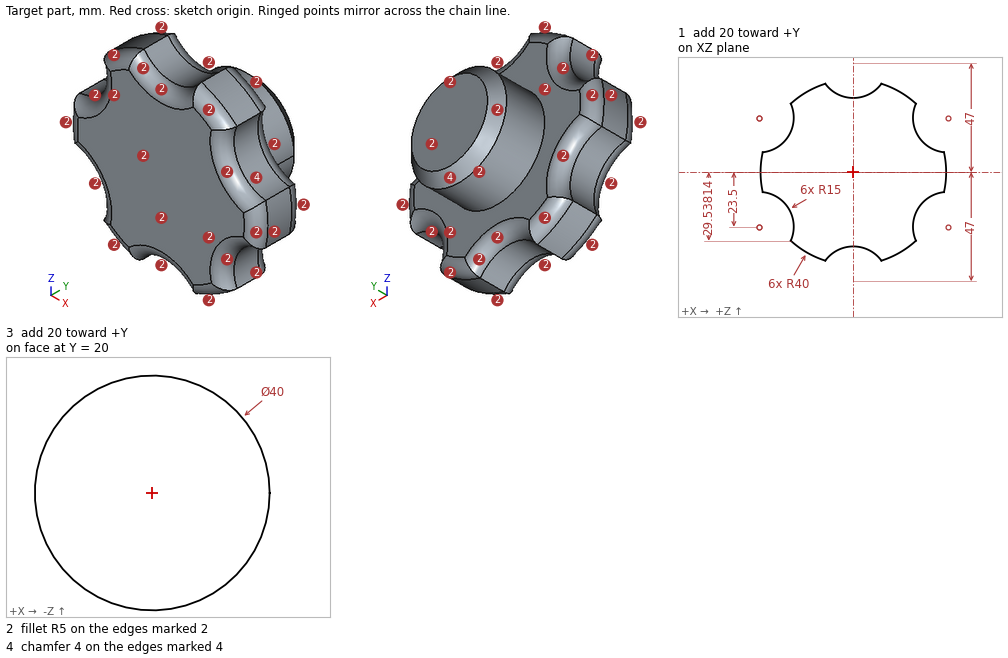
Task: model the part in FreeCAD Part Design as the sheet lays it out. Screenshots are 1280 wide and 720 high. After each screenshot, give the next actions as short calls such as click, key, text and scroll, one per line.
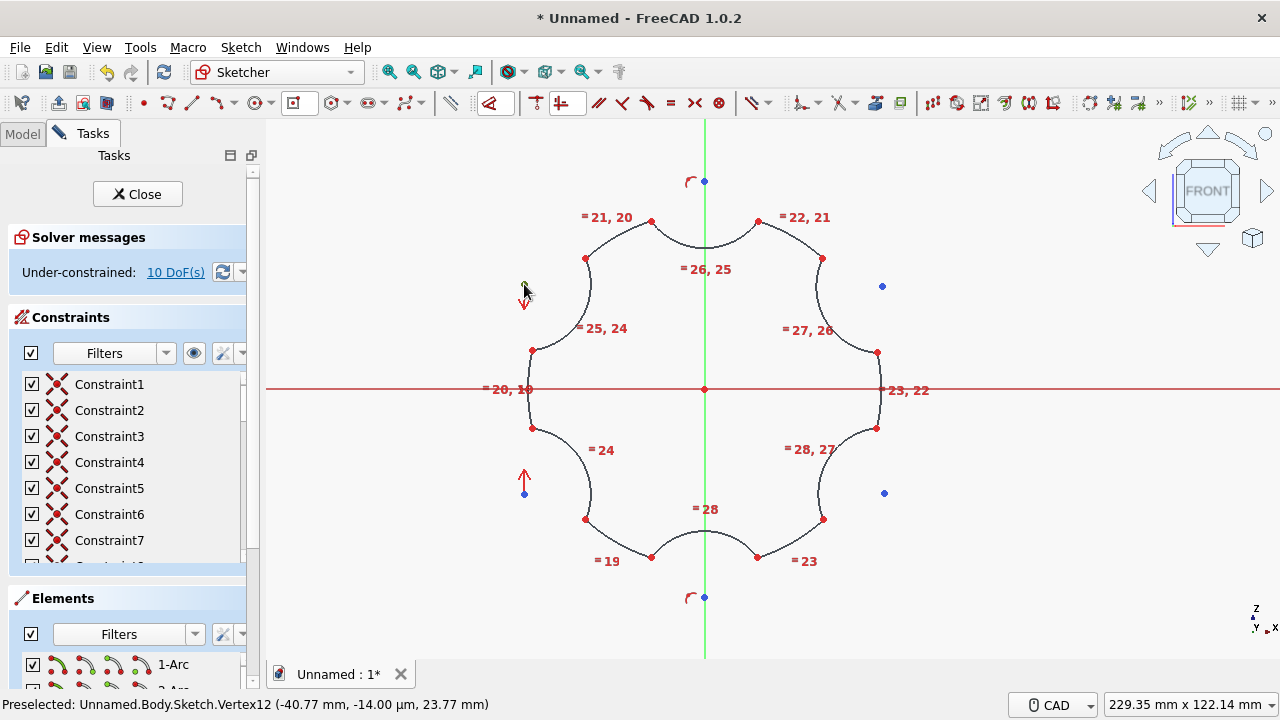
click(883, 287)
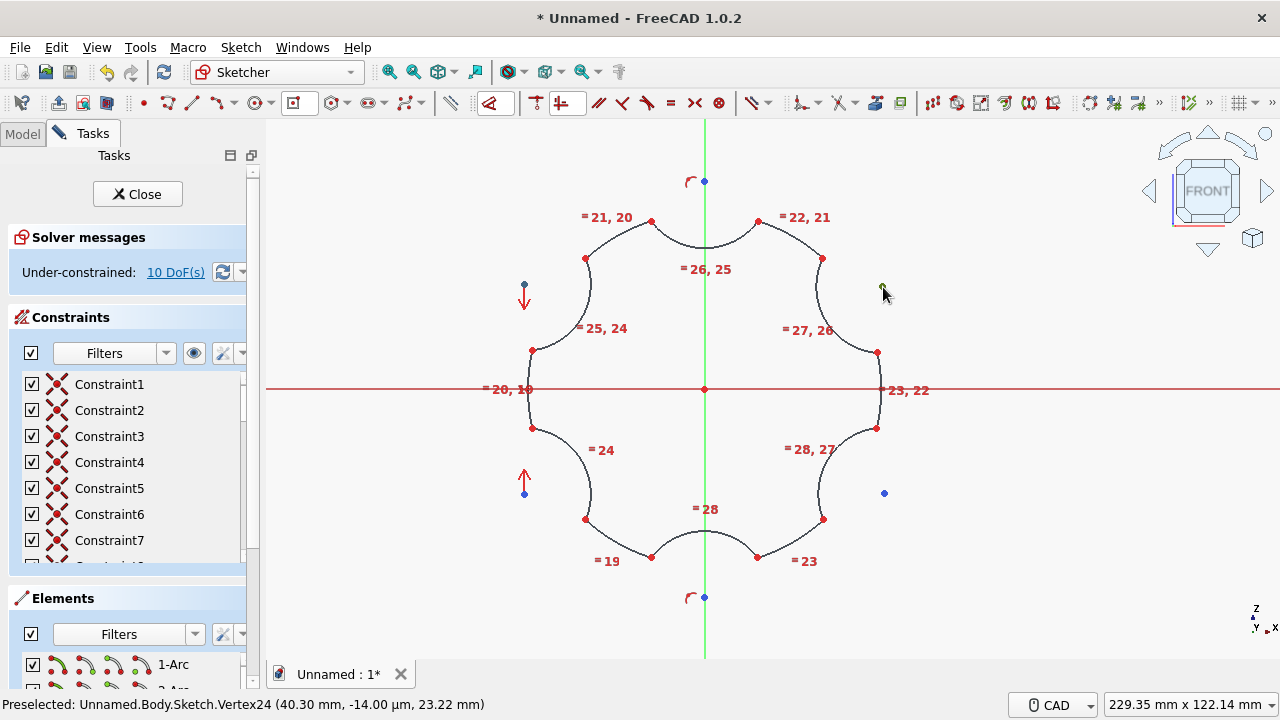
click(705, 562)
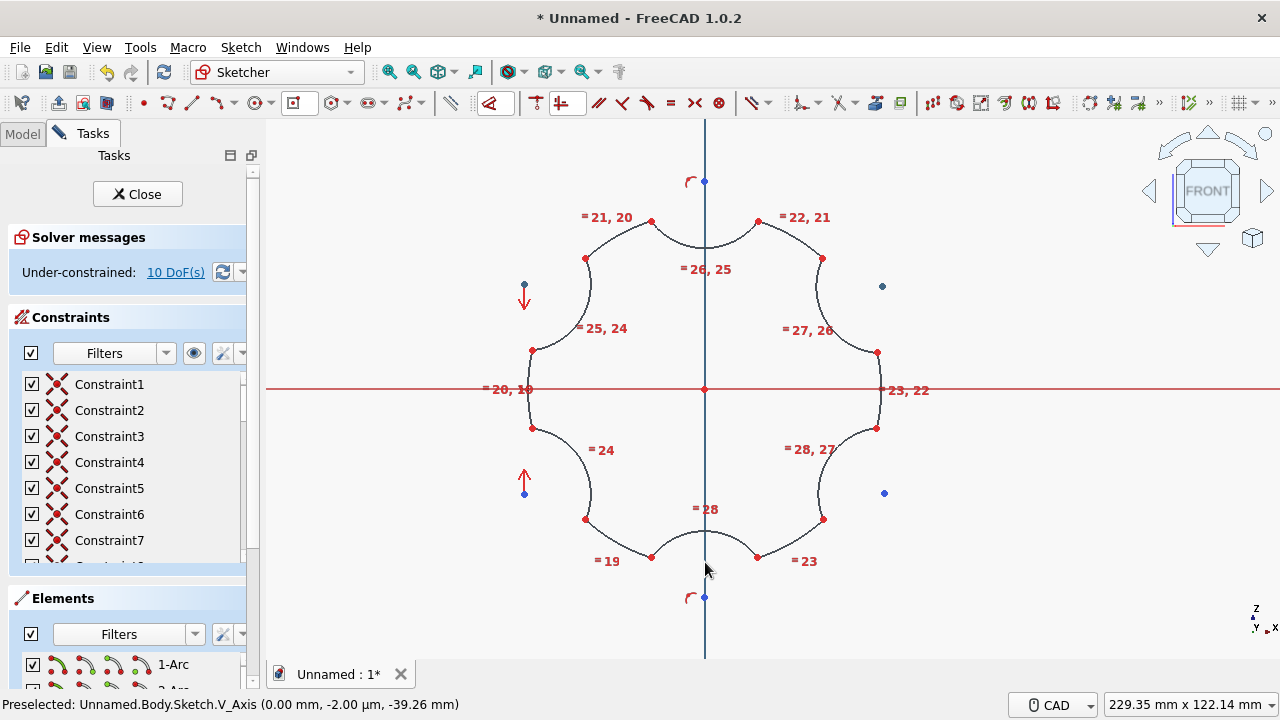
click(696, 104)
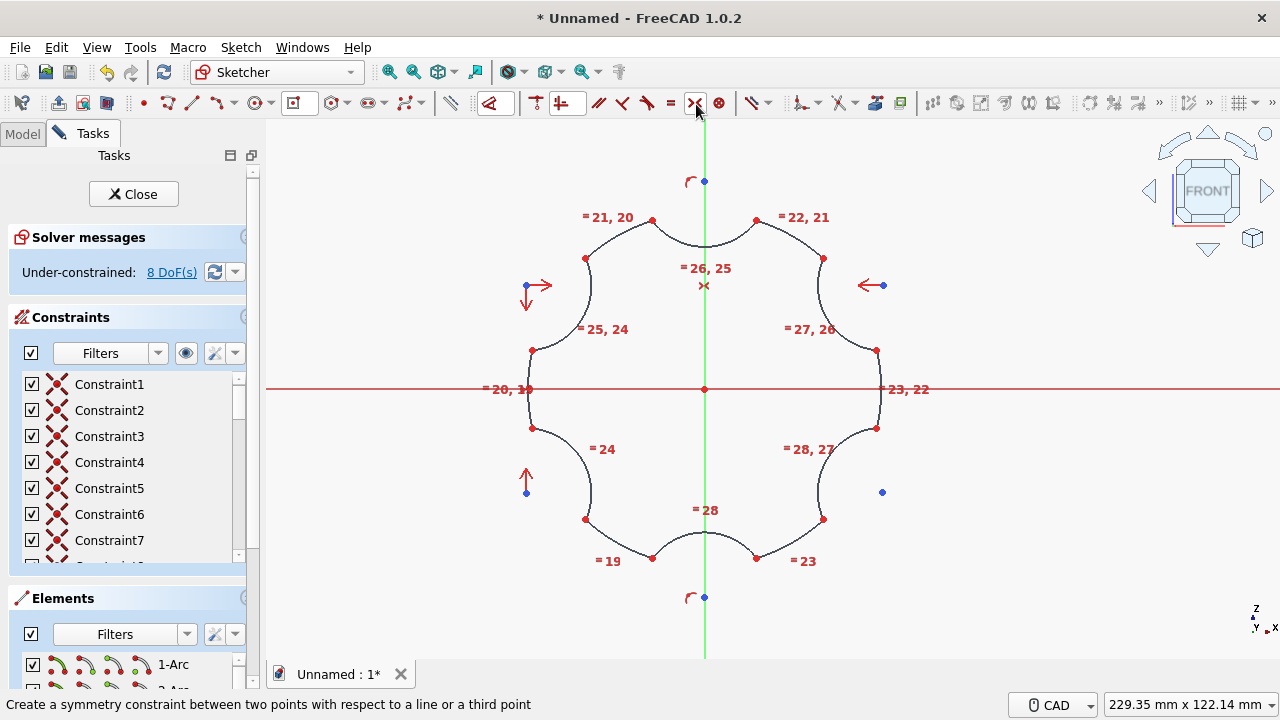
click(526, 493)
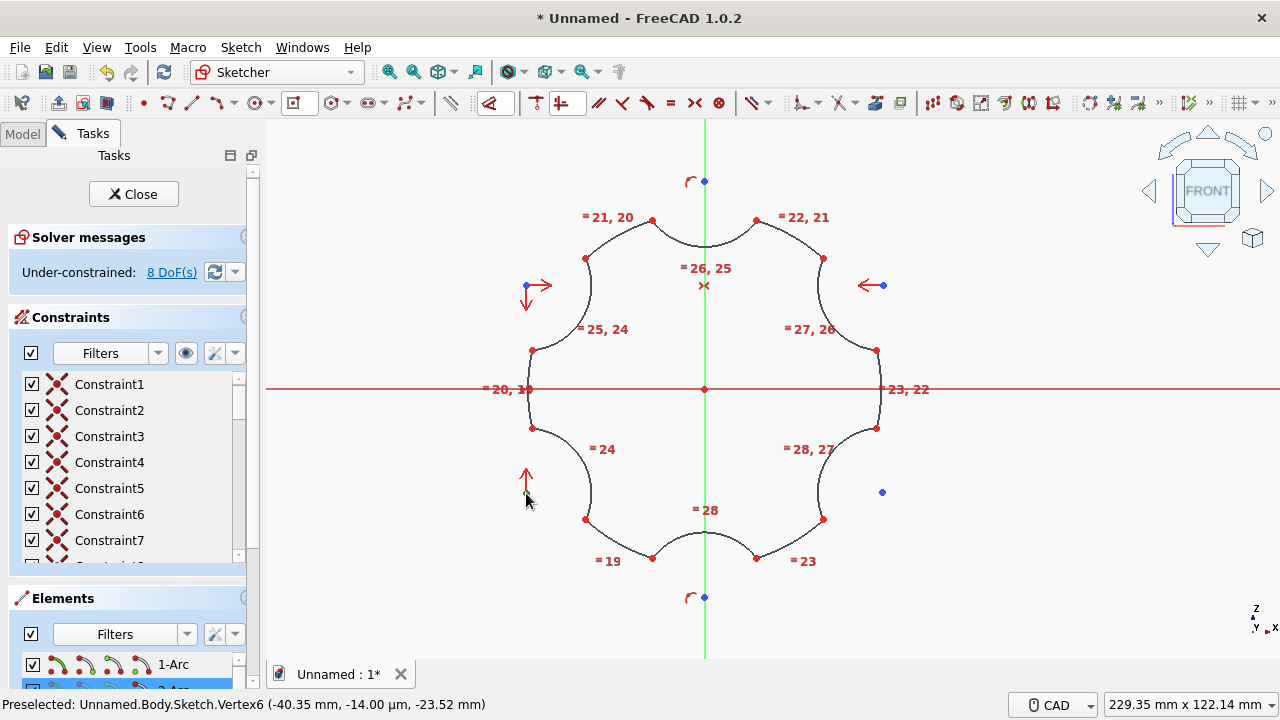
click(883, 493)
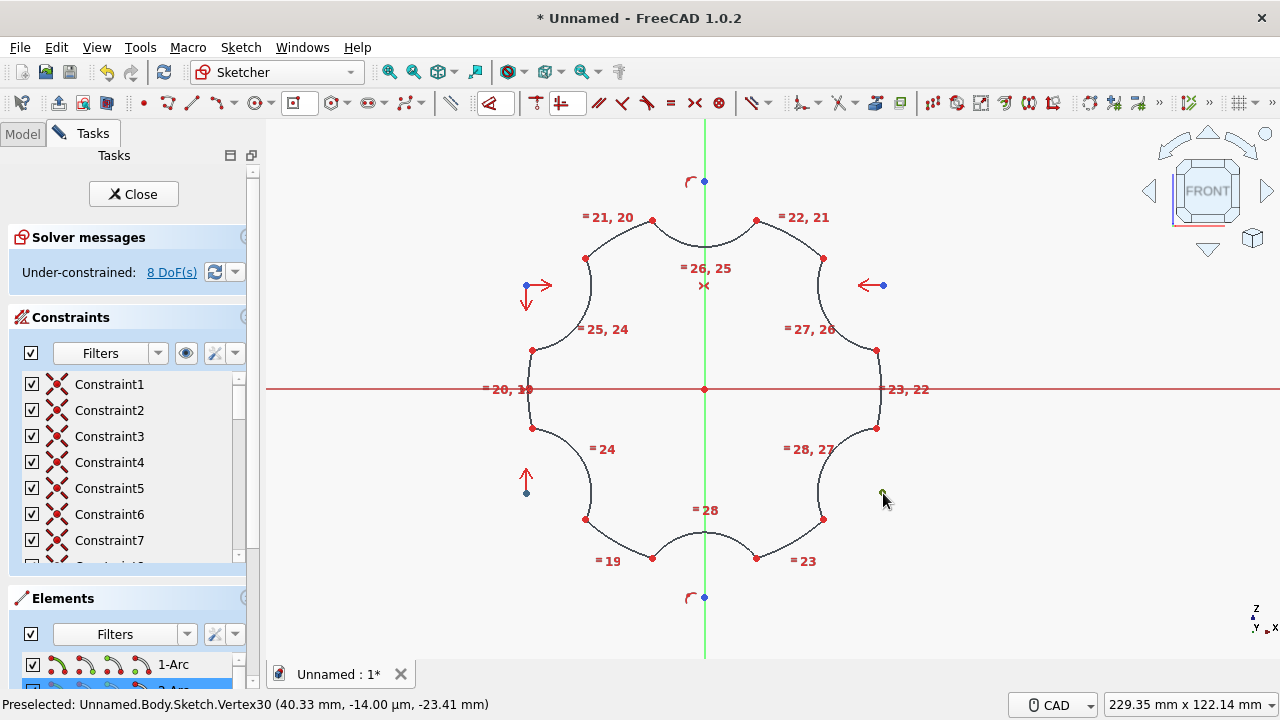
click(705, 493)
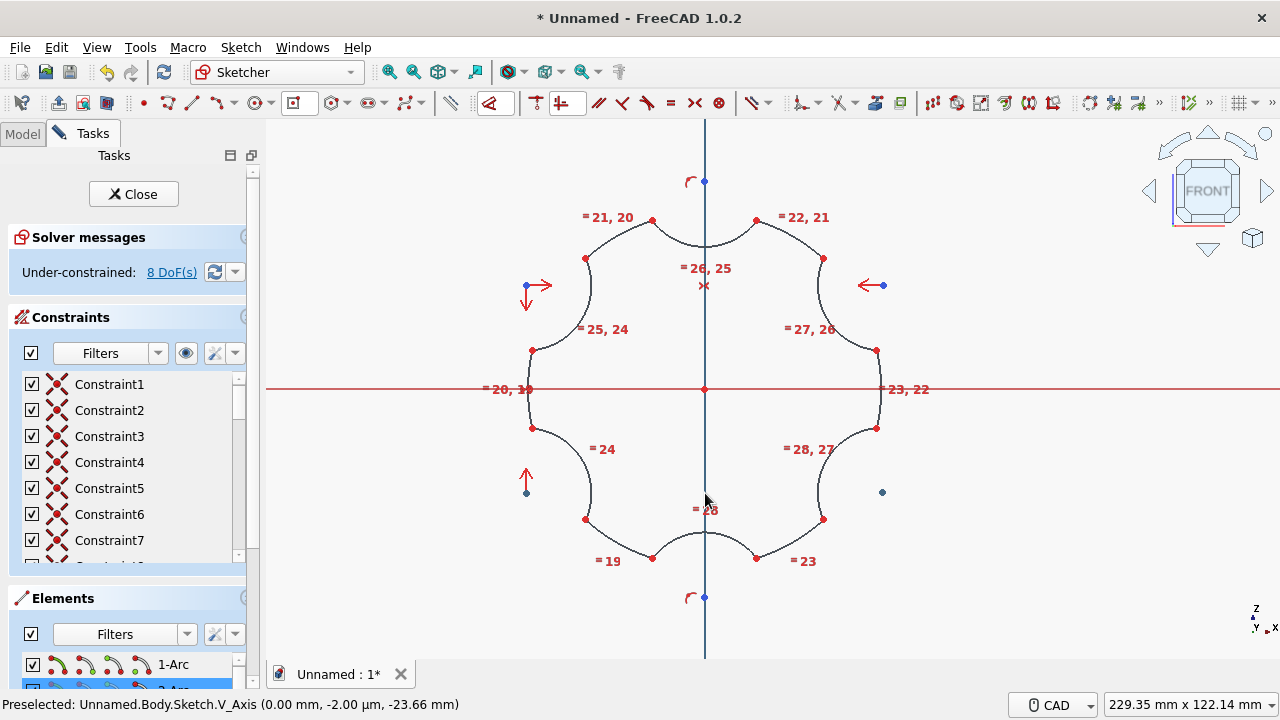
click(696, 104)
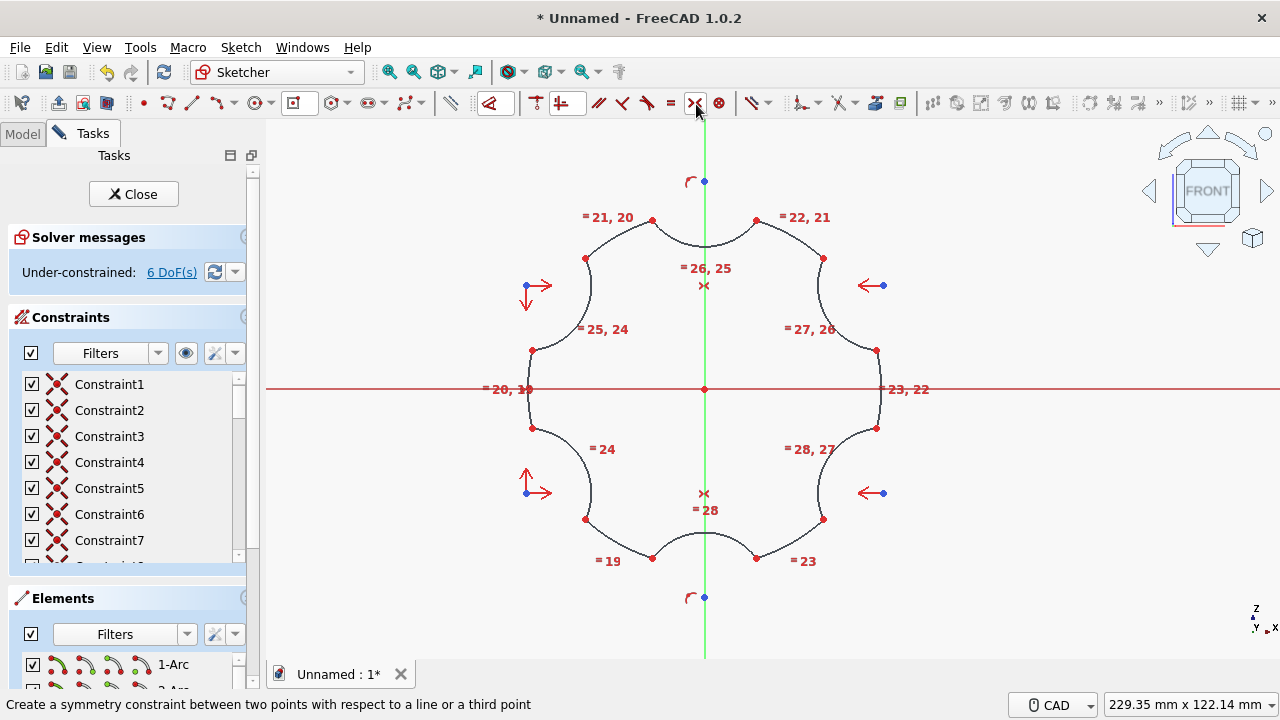
click(604, 534)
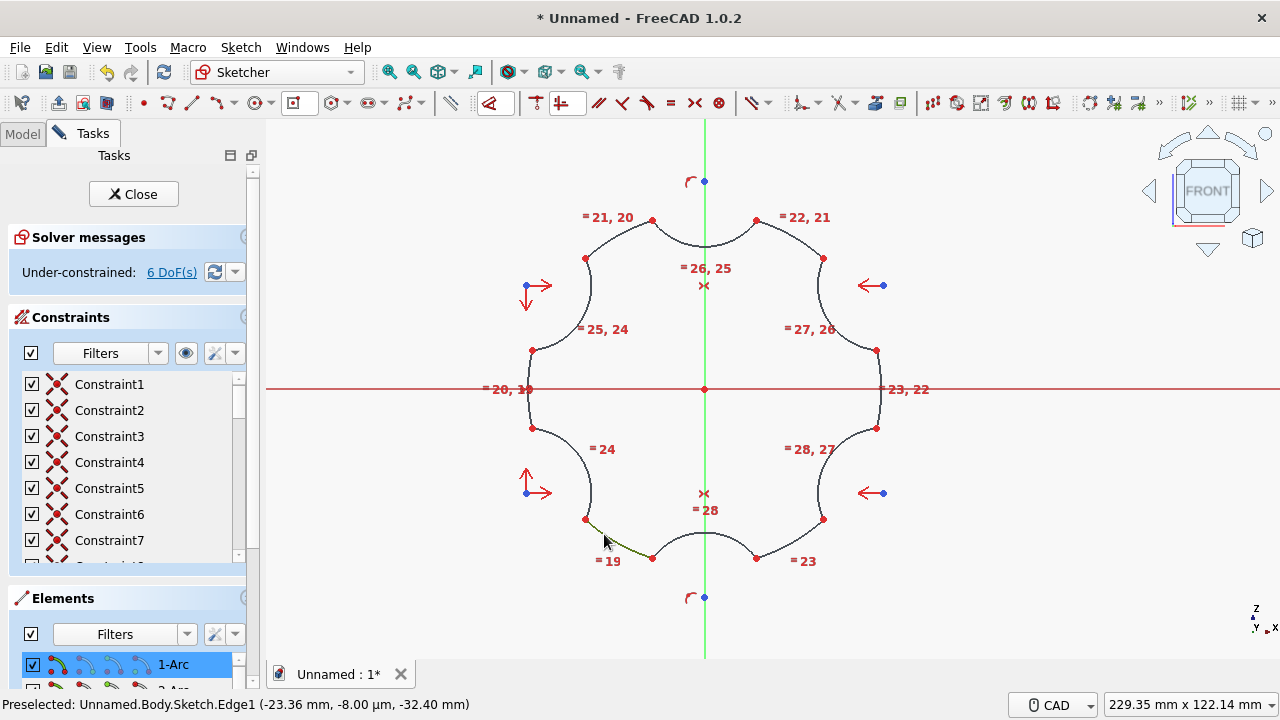
key(k)
key(r)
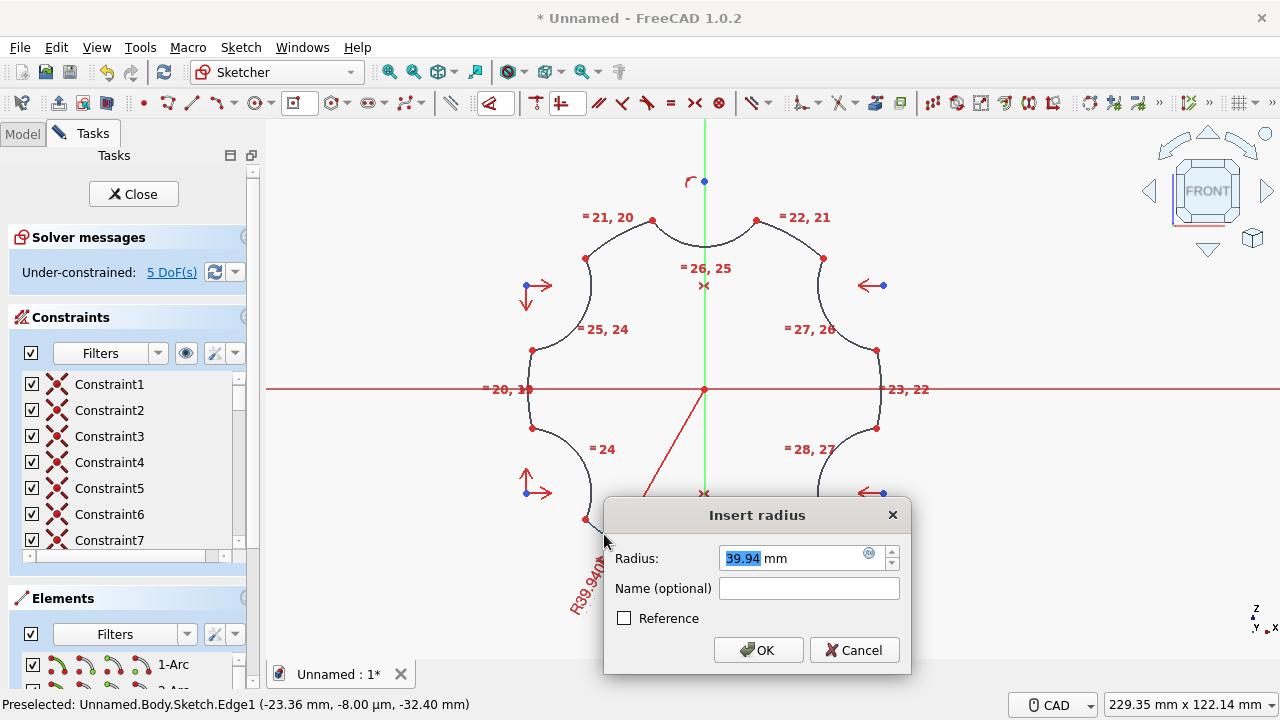
text(40)
key(Return)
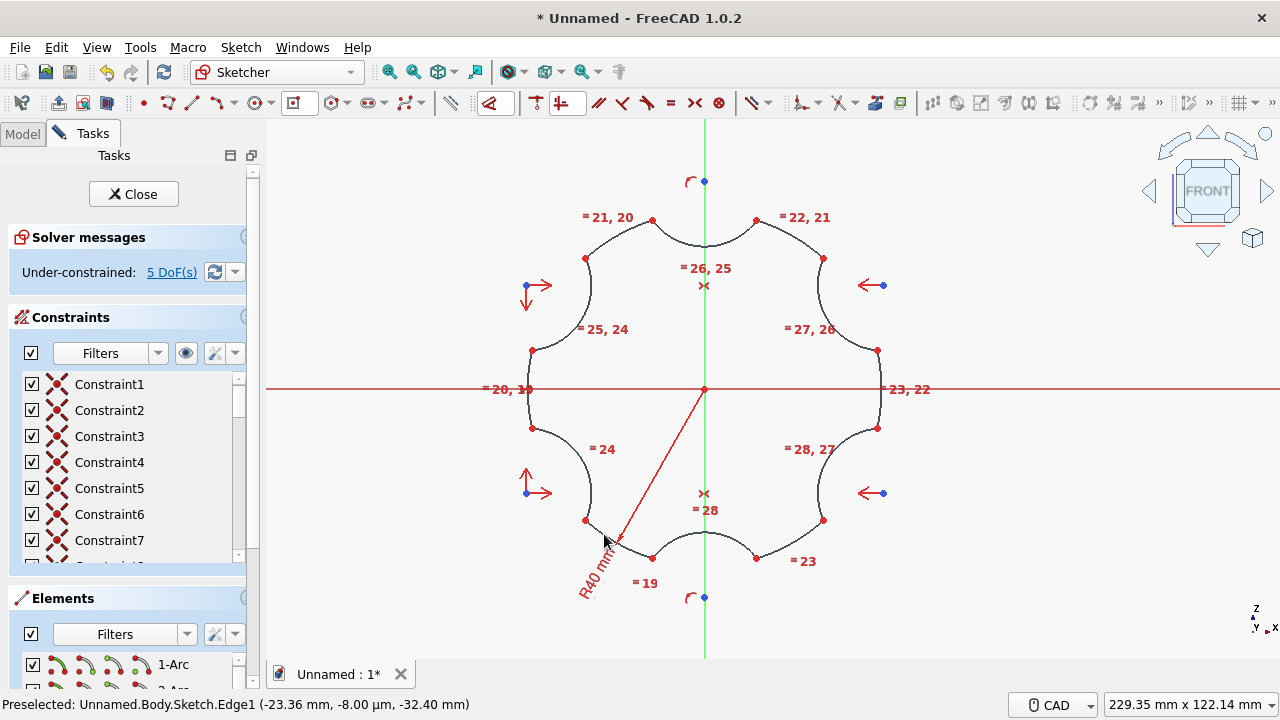
click(591, 484)